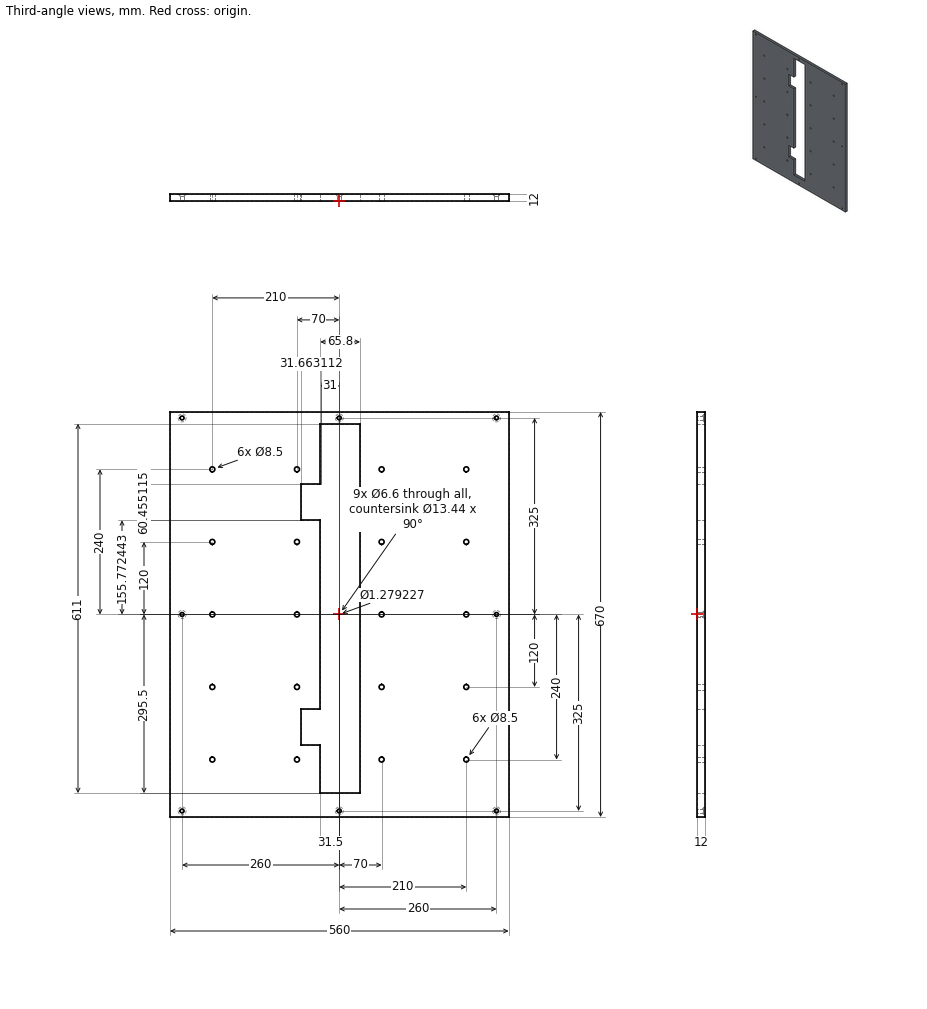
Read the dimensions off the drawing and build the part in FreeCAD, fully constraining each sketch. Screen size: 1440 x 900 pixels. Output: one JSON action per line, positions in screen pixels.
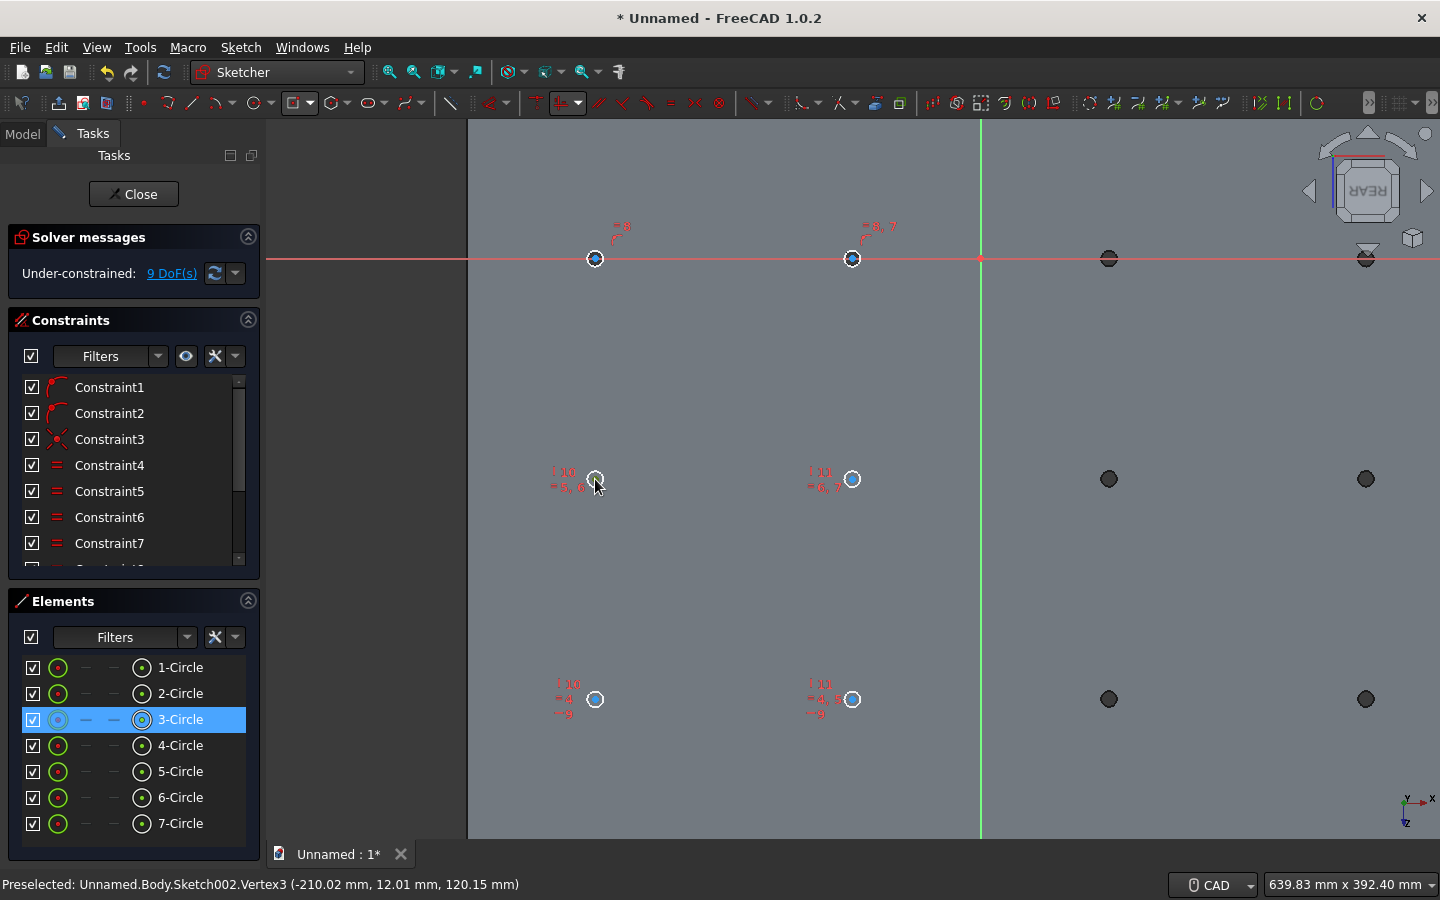
{"action": "left_click", "coordinate": [852, 479]}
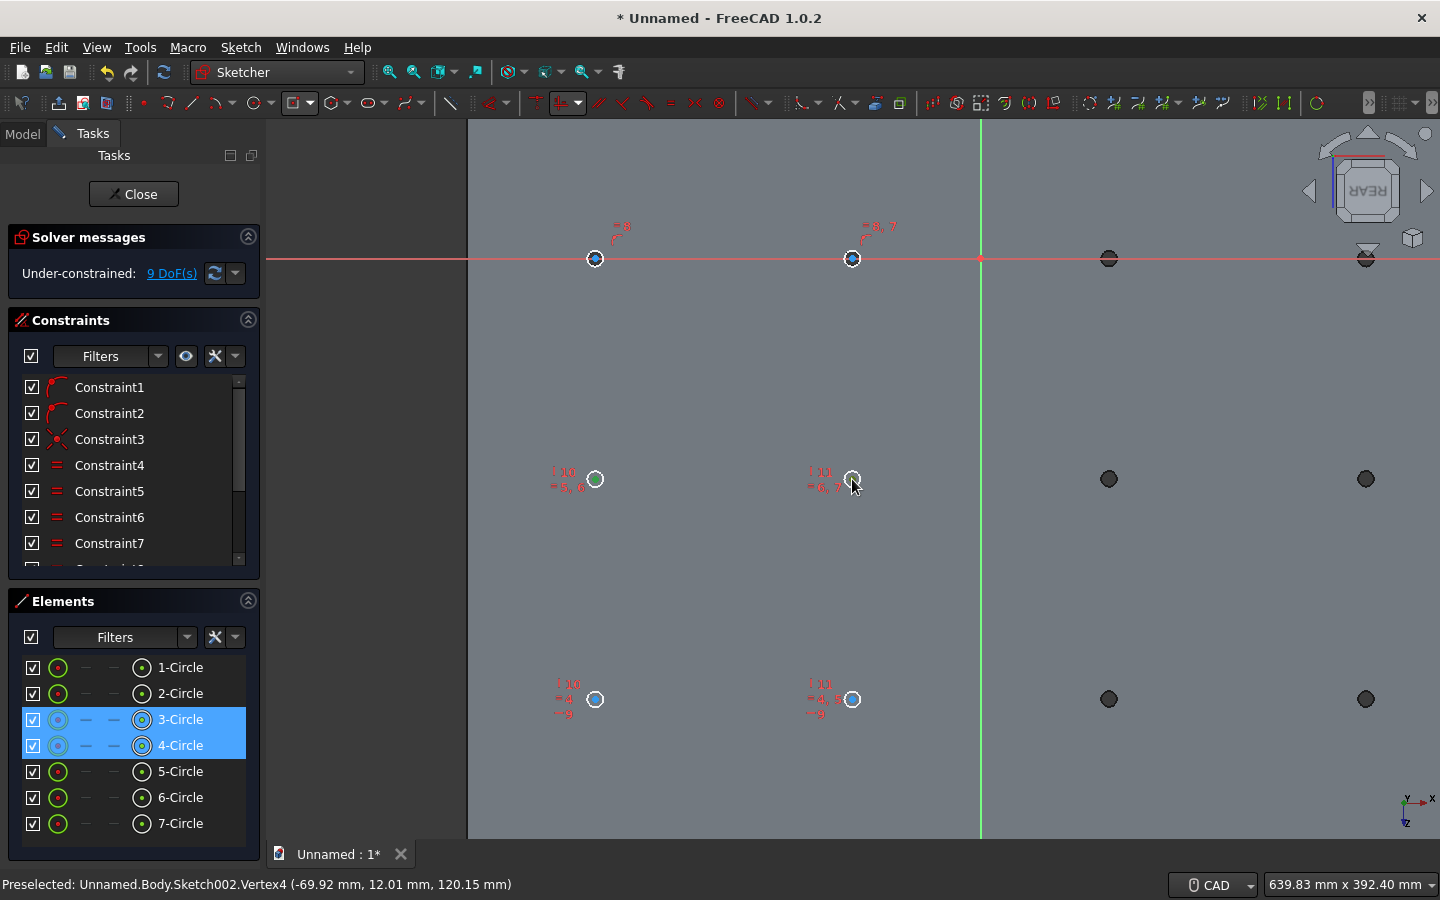
{"action": "left_click", "coordinate": [580, 104]}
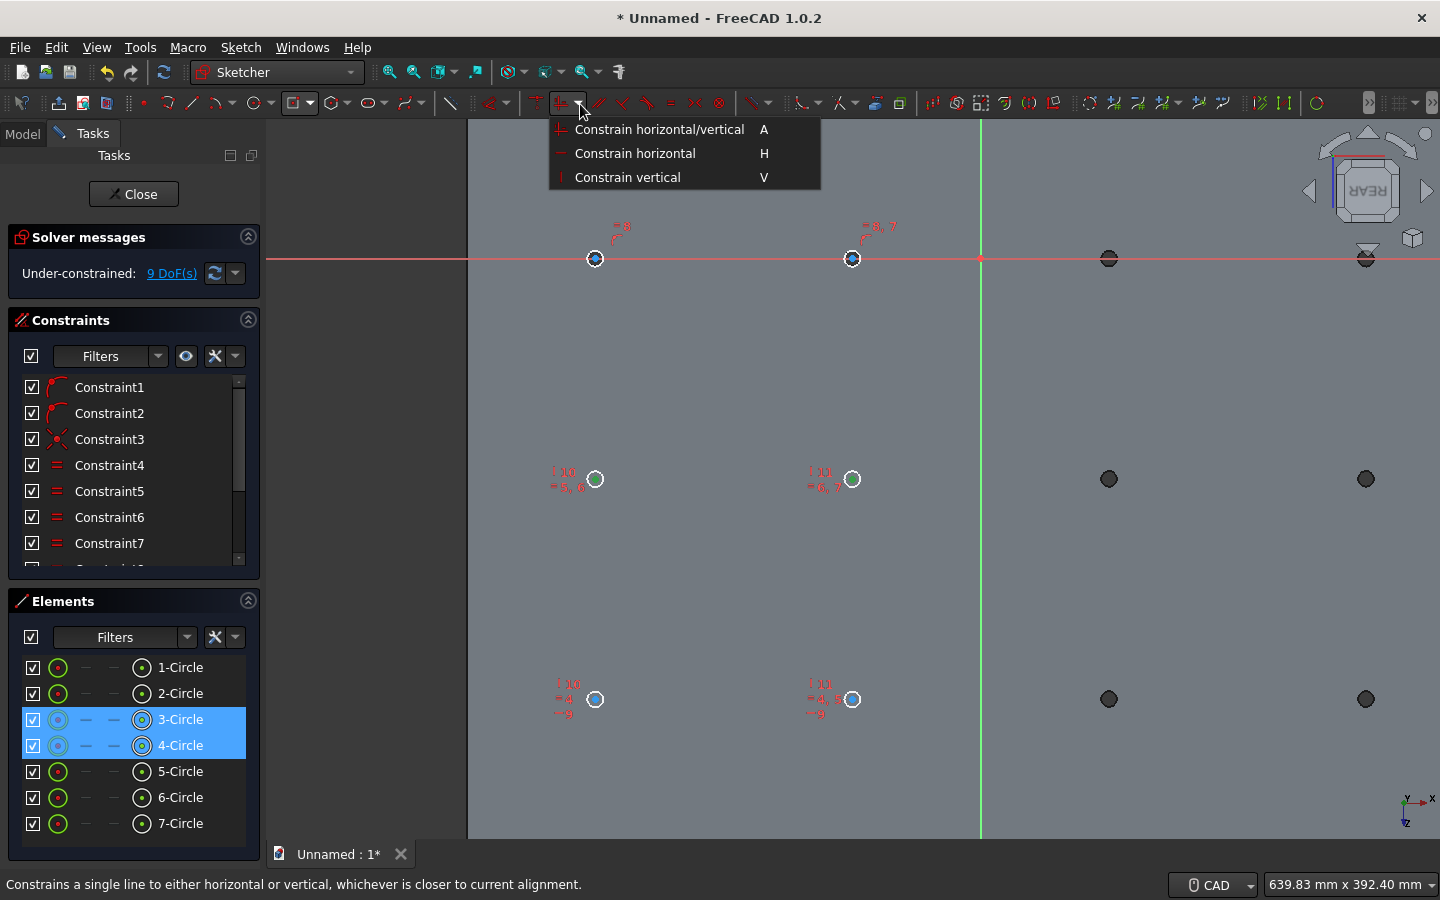
{"action": "left_click", "coordinate": [685, 153]}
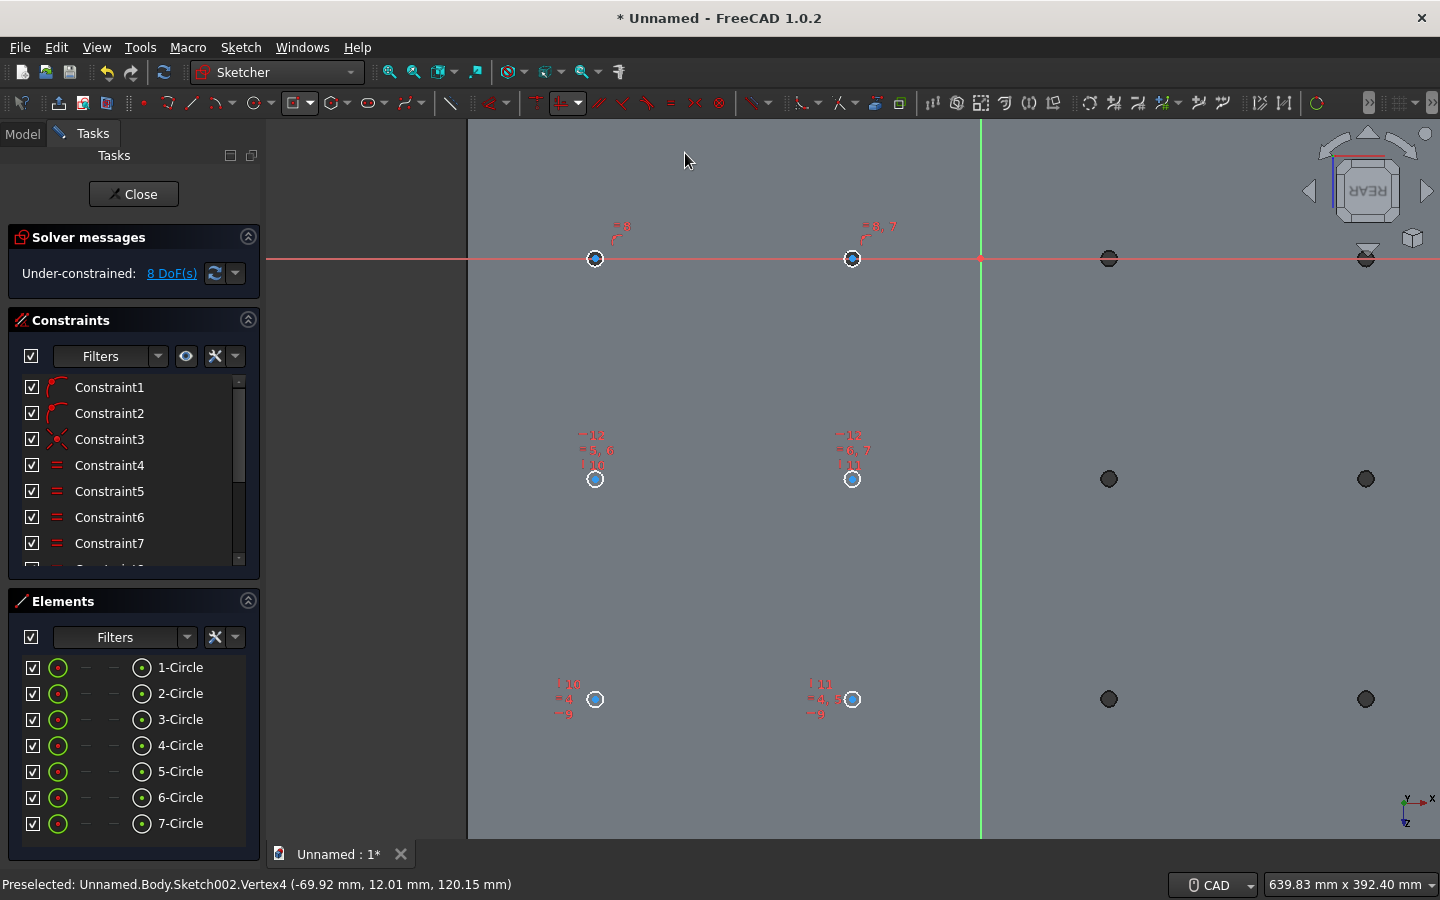
{"action": "left_click", "coordinate": [852, 479]}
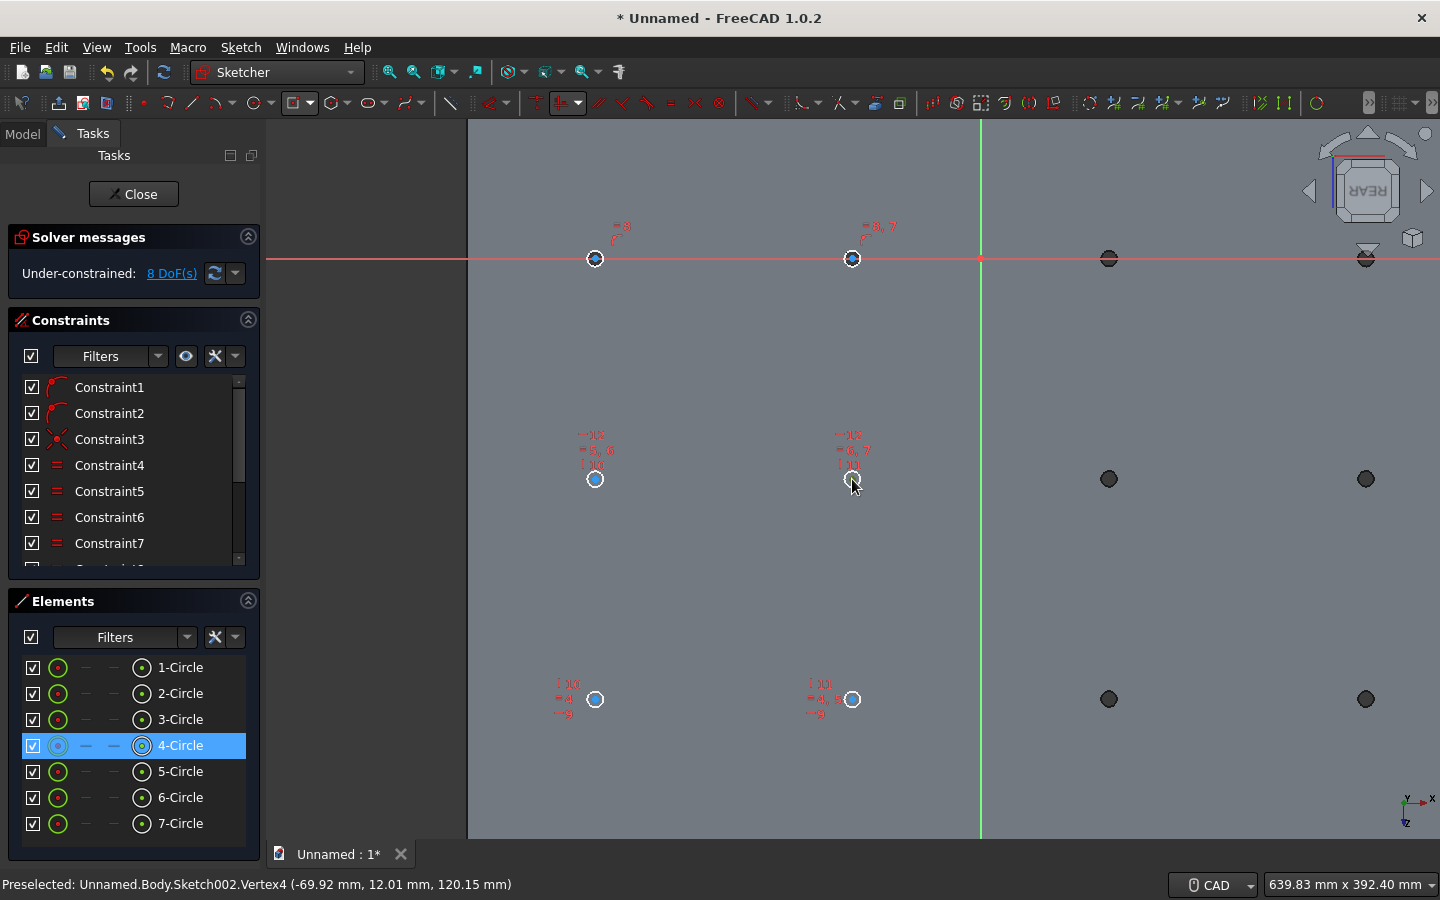
{"action": "left_click", "coordinate": [852, 259]}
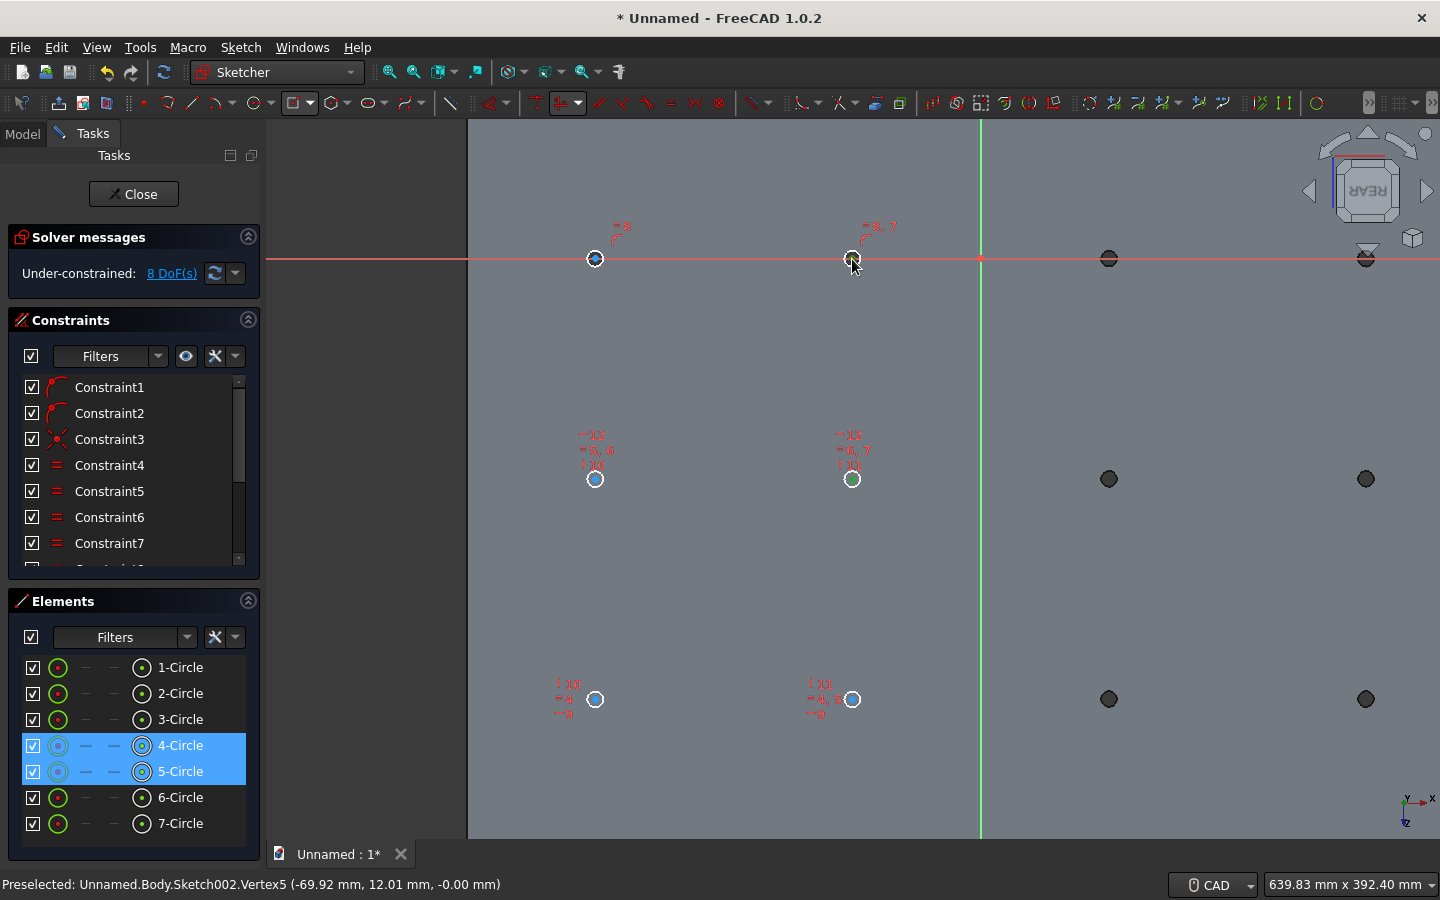
{"action": "left_click", "coordinate": [580, 104]}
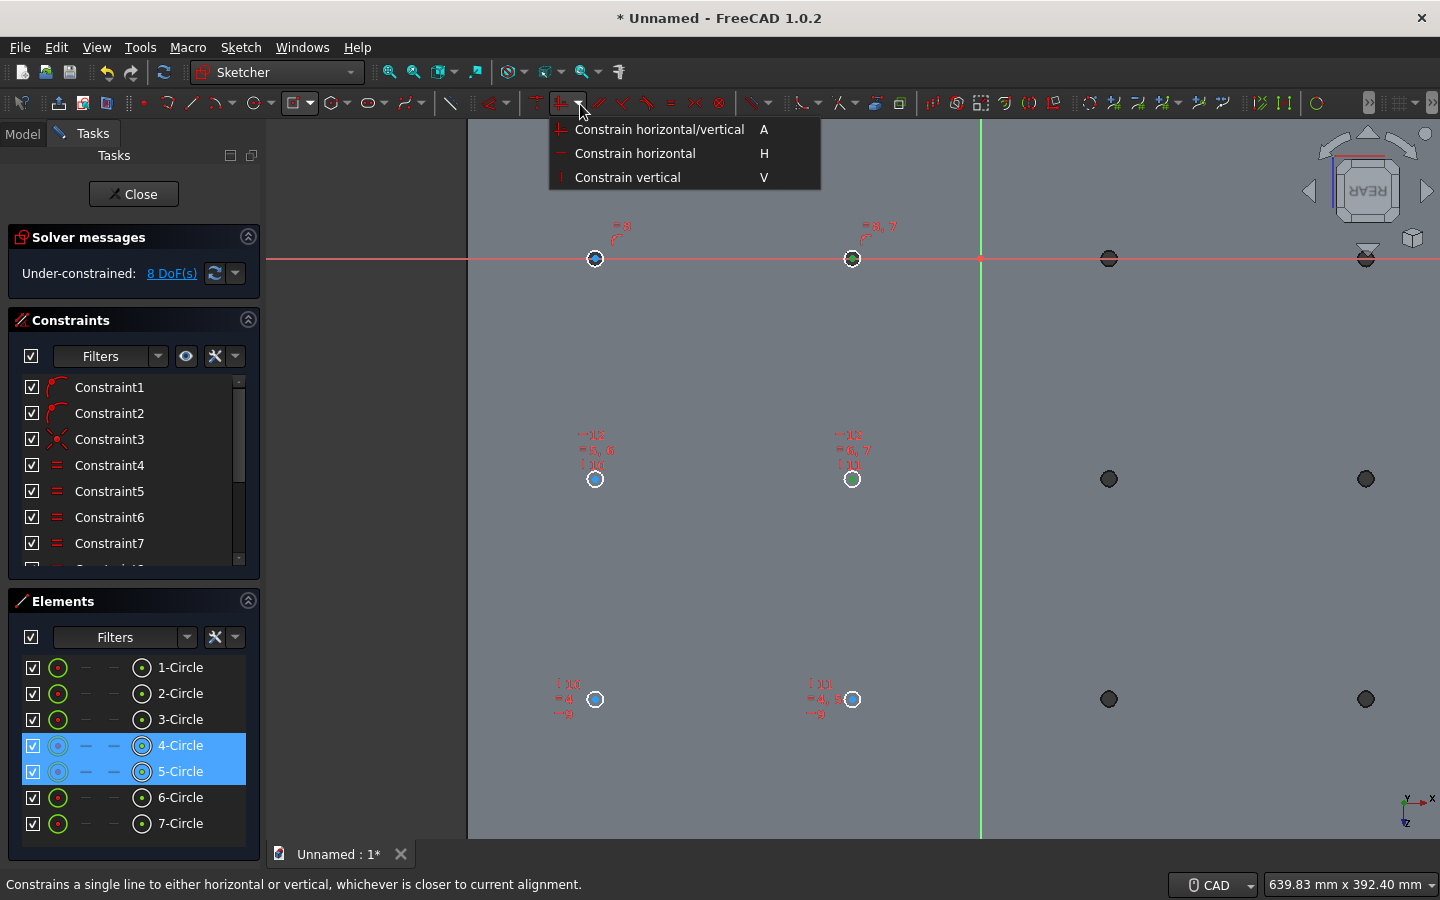
{"action": "left_click", "coordinate": [685, 177]}